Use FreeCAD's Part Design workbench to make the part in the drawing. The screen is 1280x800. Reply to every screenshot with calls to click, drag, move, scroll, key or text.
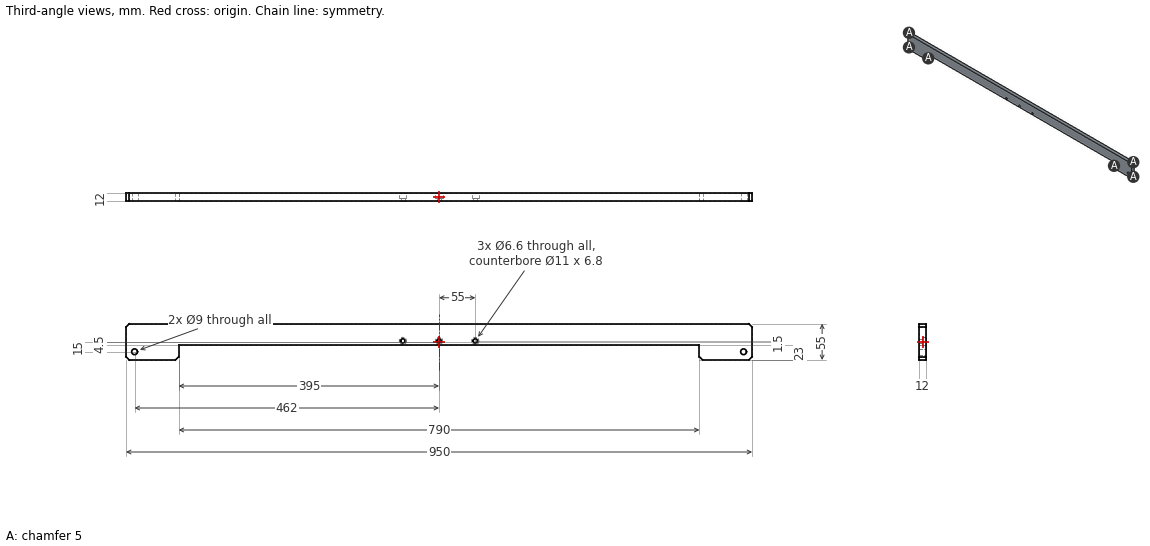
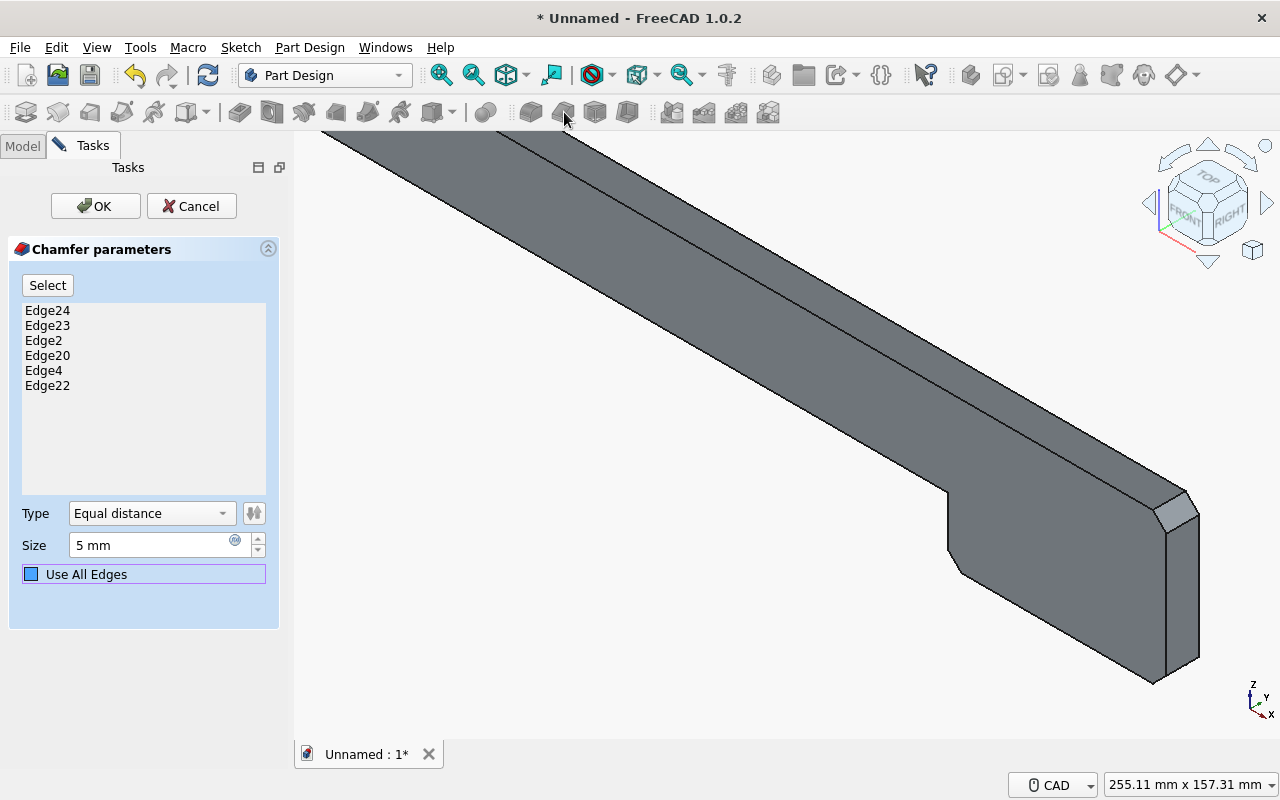
click(96, 206)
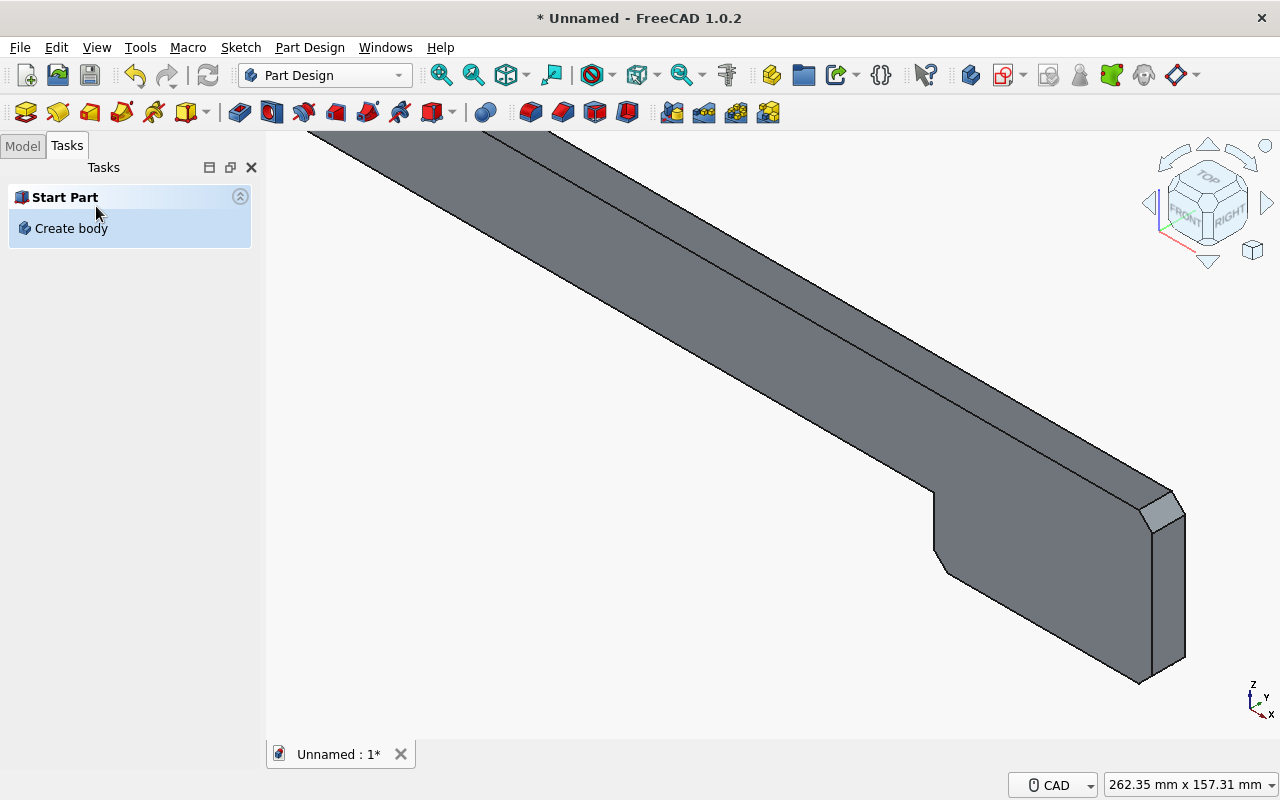
click(442, 76)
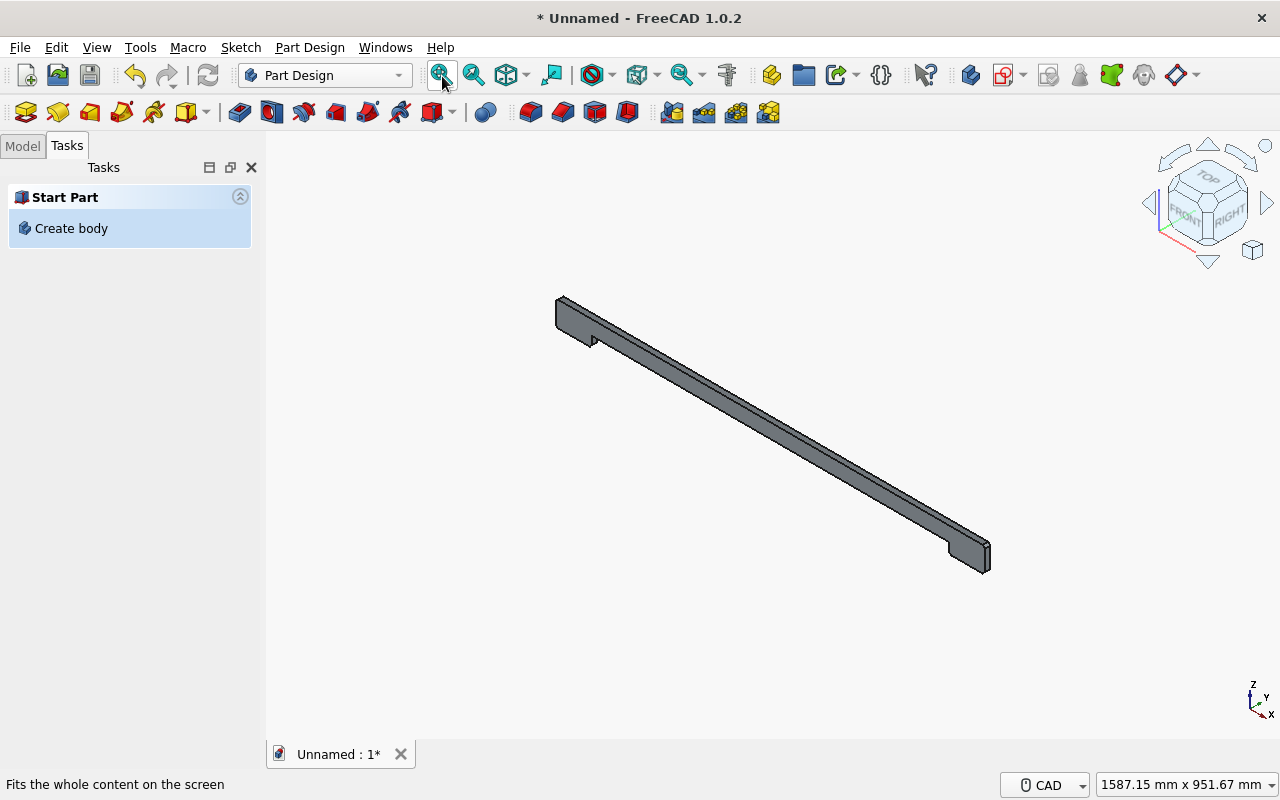
click(954, 538)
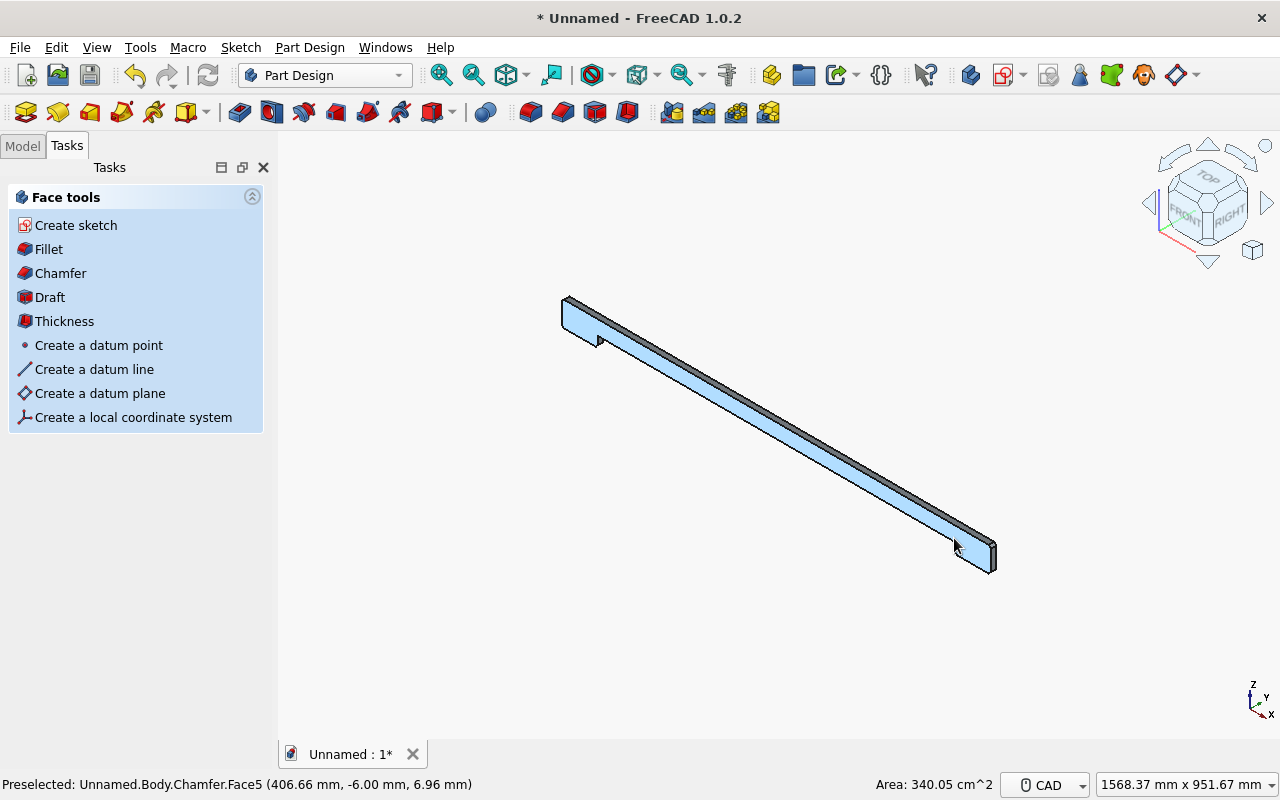
click(1004, 76)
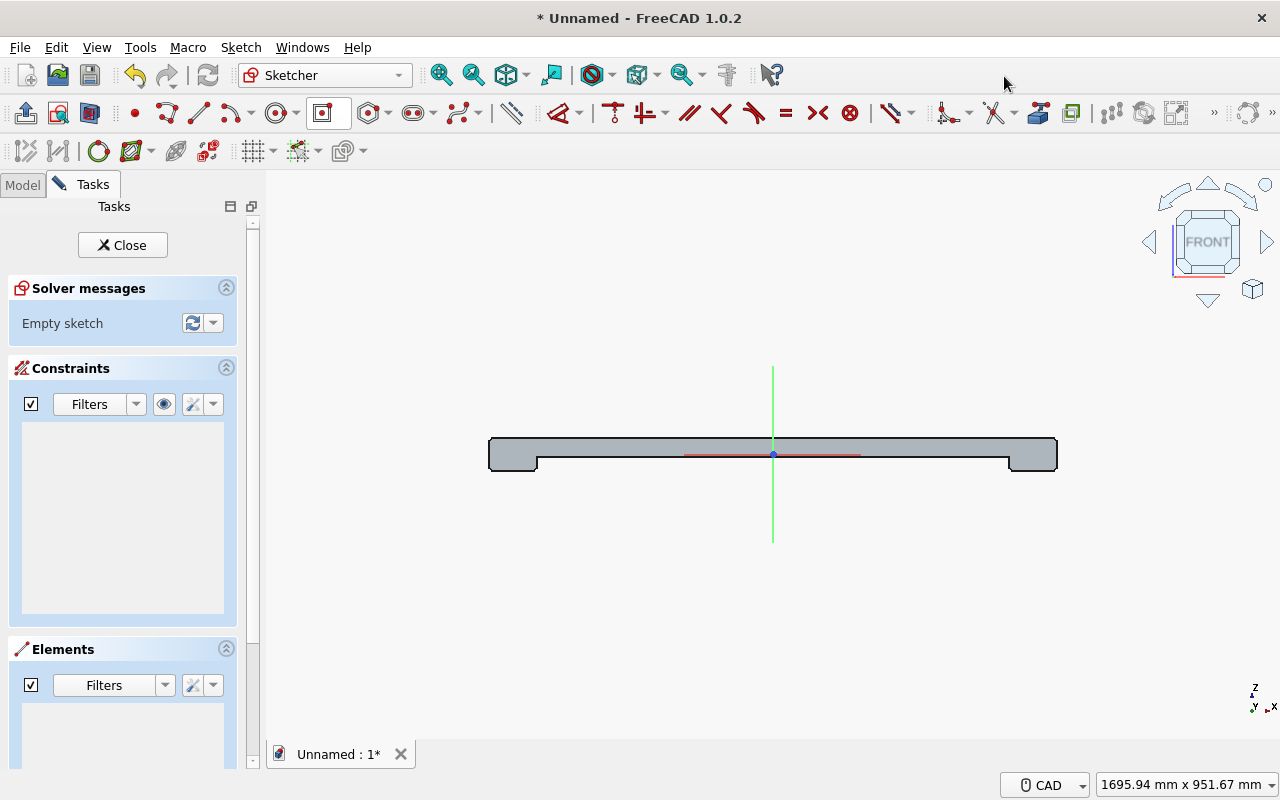
key(g)
key(c)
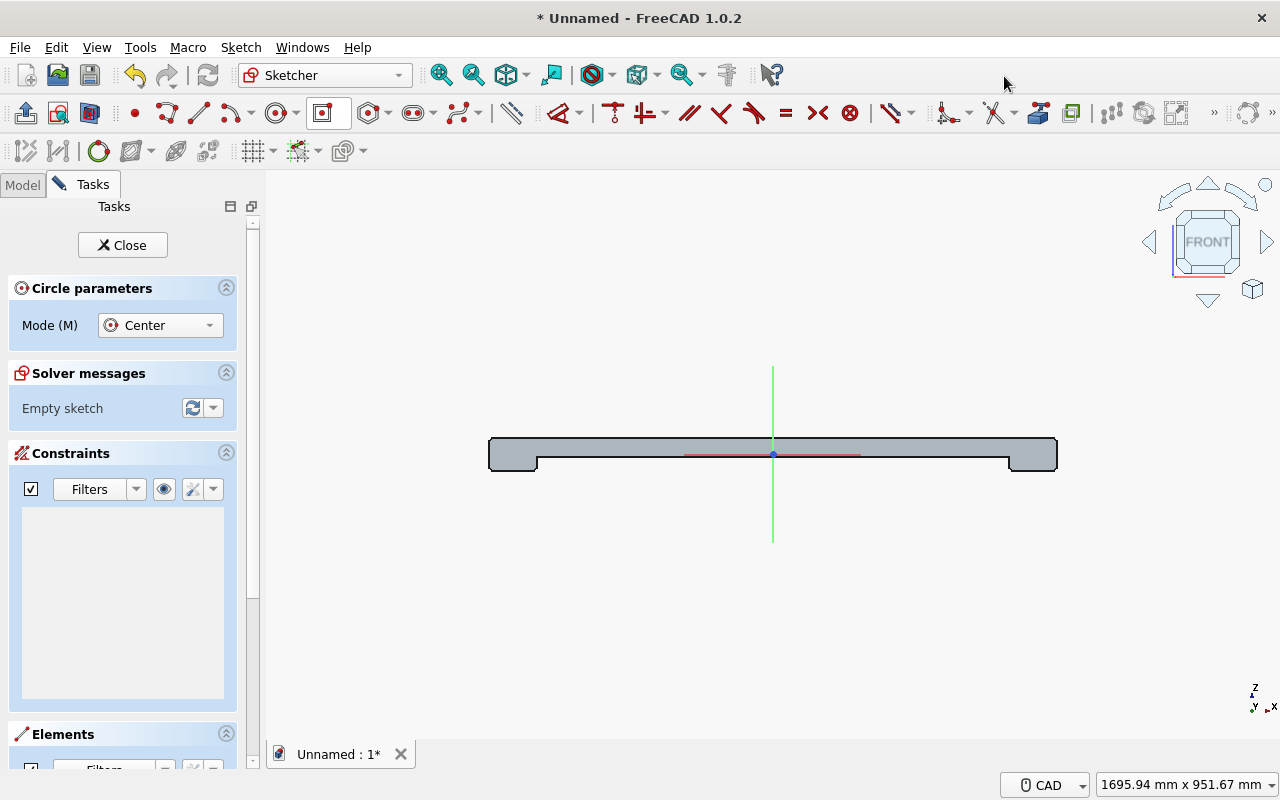
scroll(497, 463, up, 11)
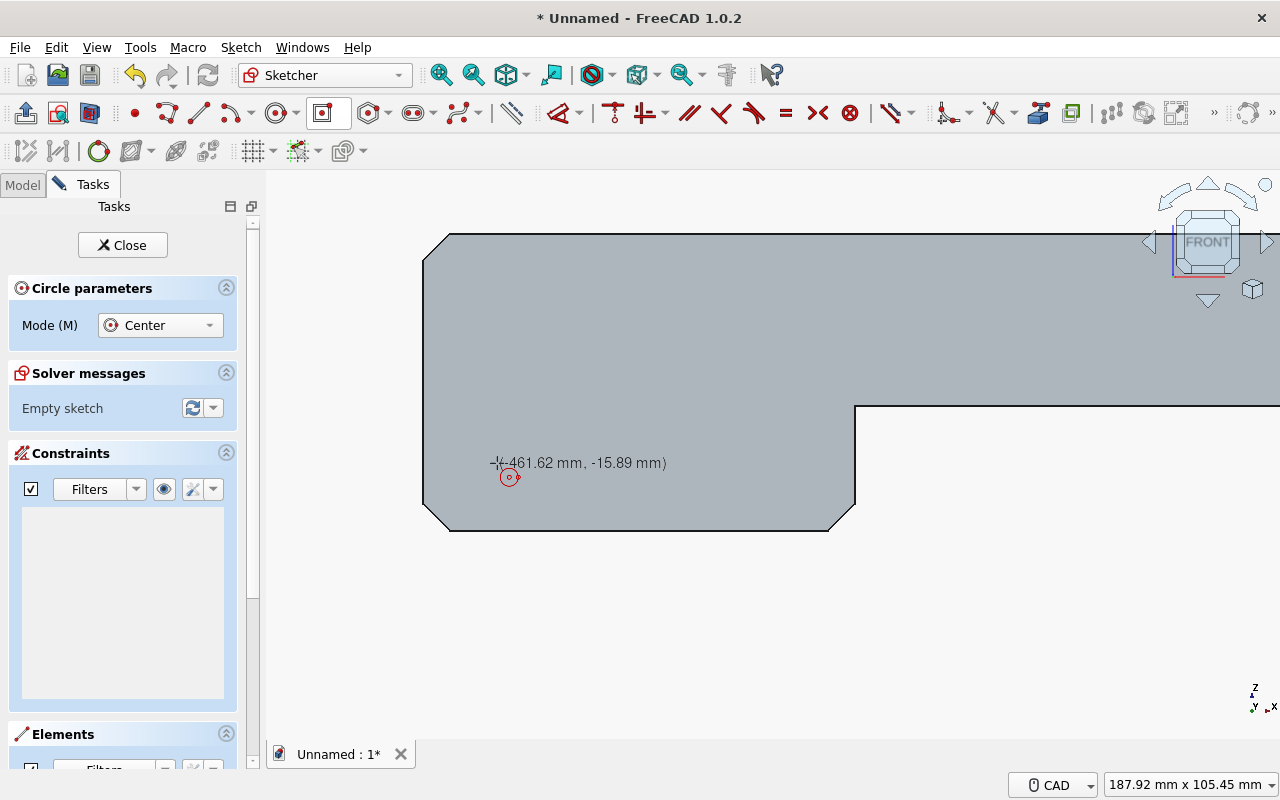
scroll(420, 457, down, 11)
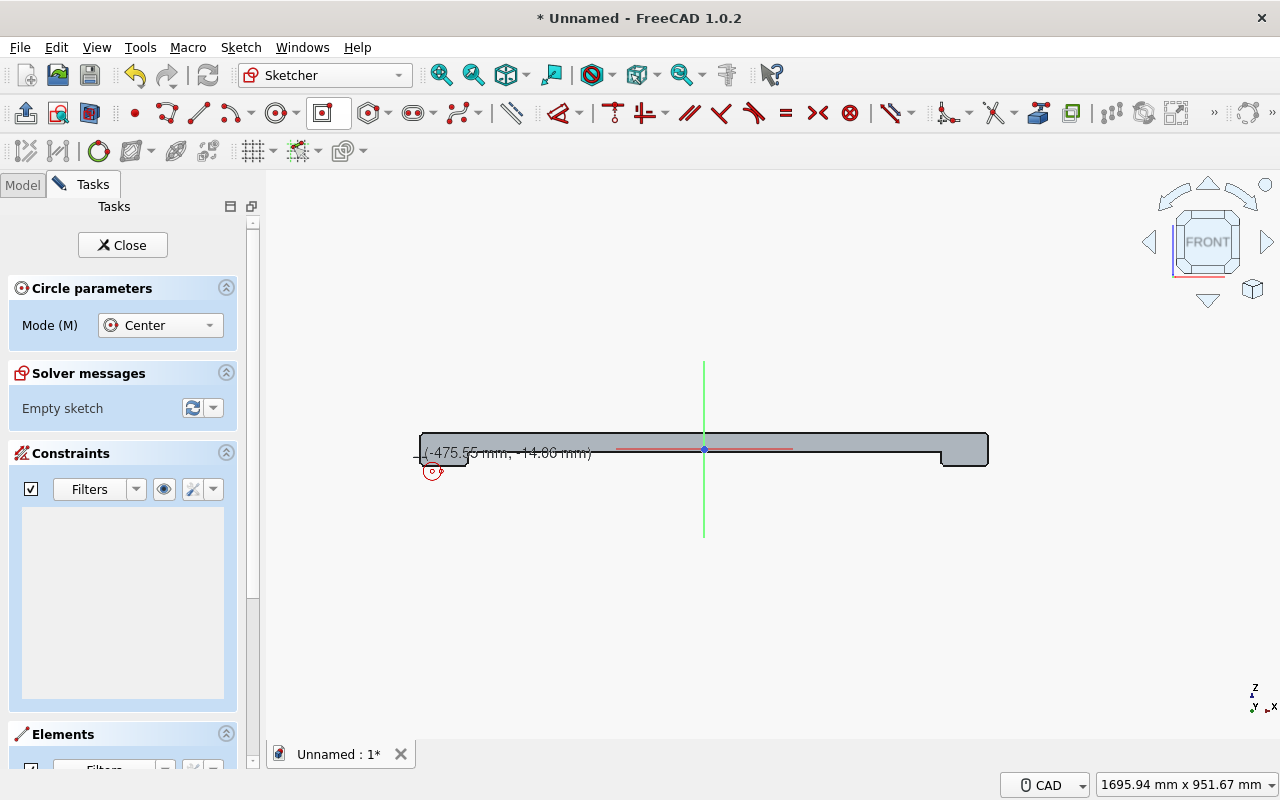
scroll(428, 458, up, 3)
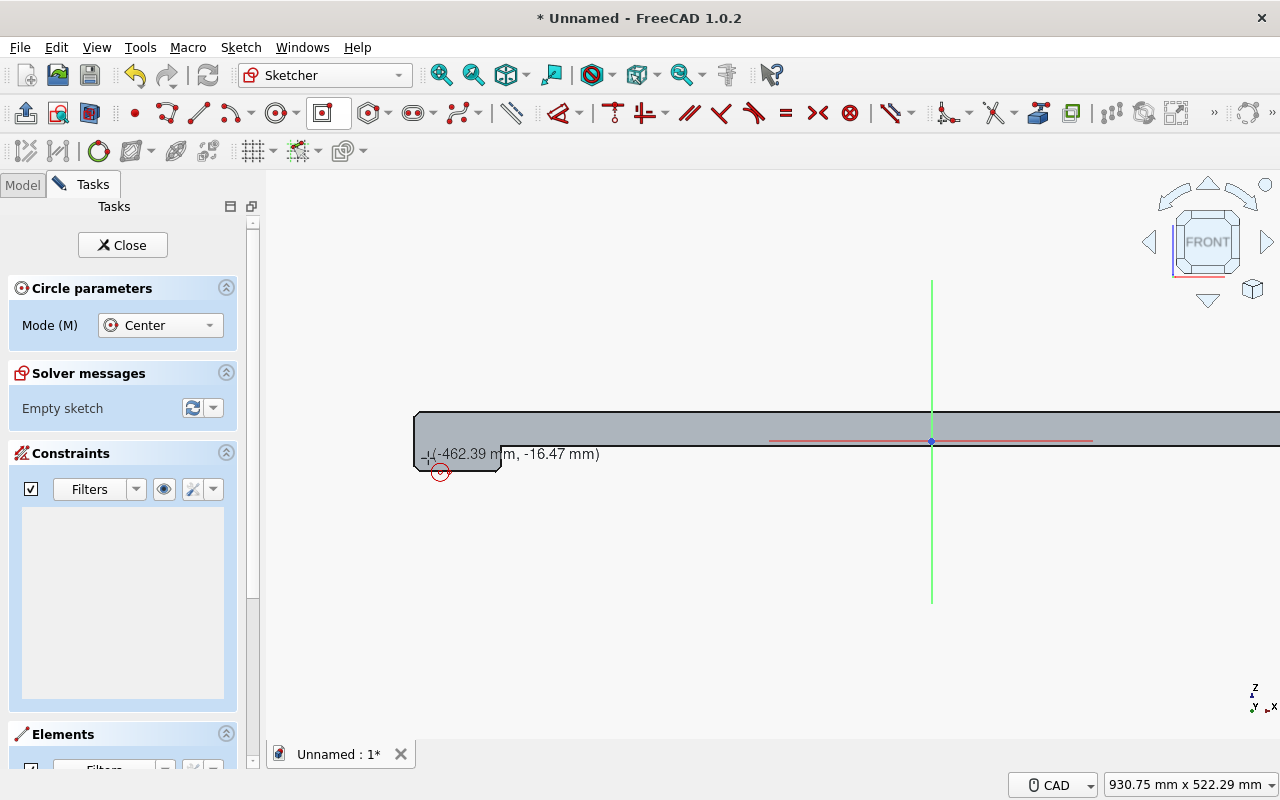
click(428, 458)
move(432, 461)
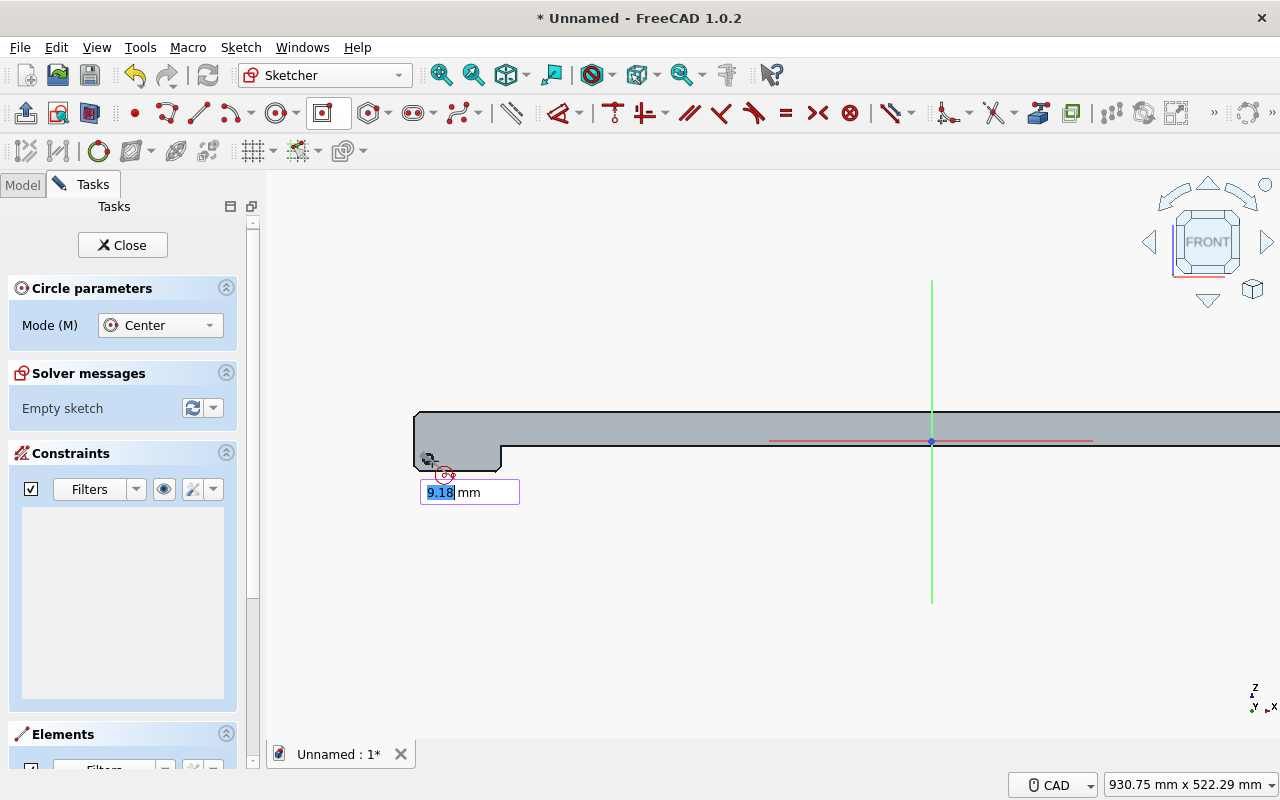
text(9)
key(Return)